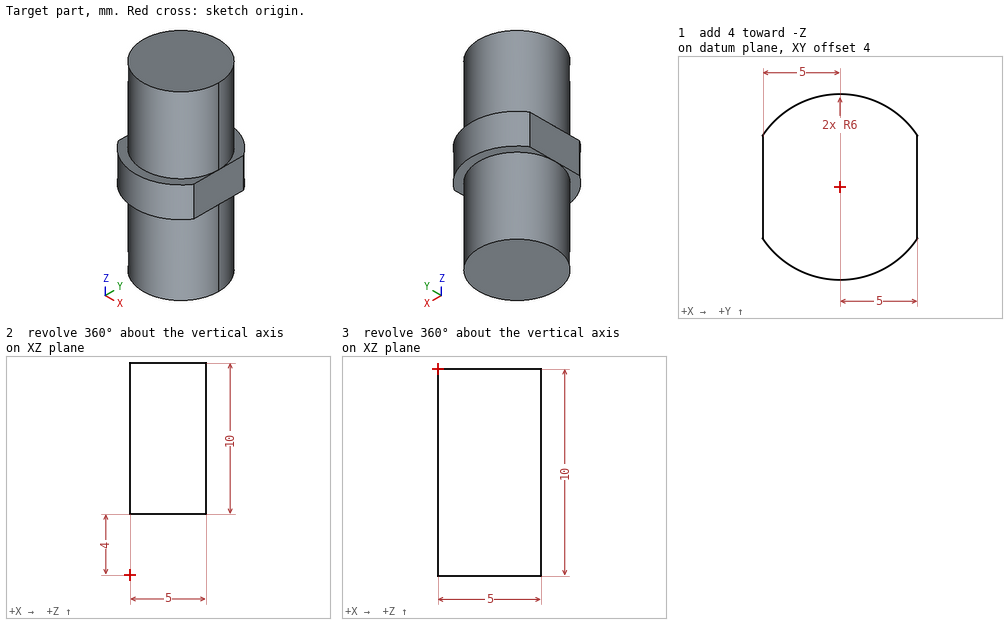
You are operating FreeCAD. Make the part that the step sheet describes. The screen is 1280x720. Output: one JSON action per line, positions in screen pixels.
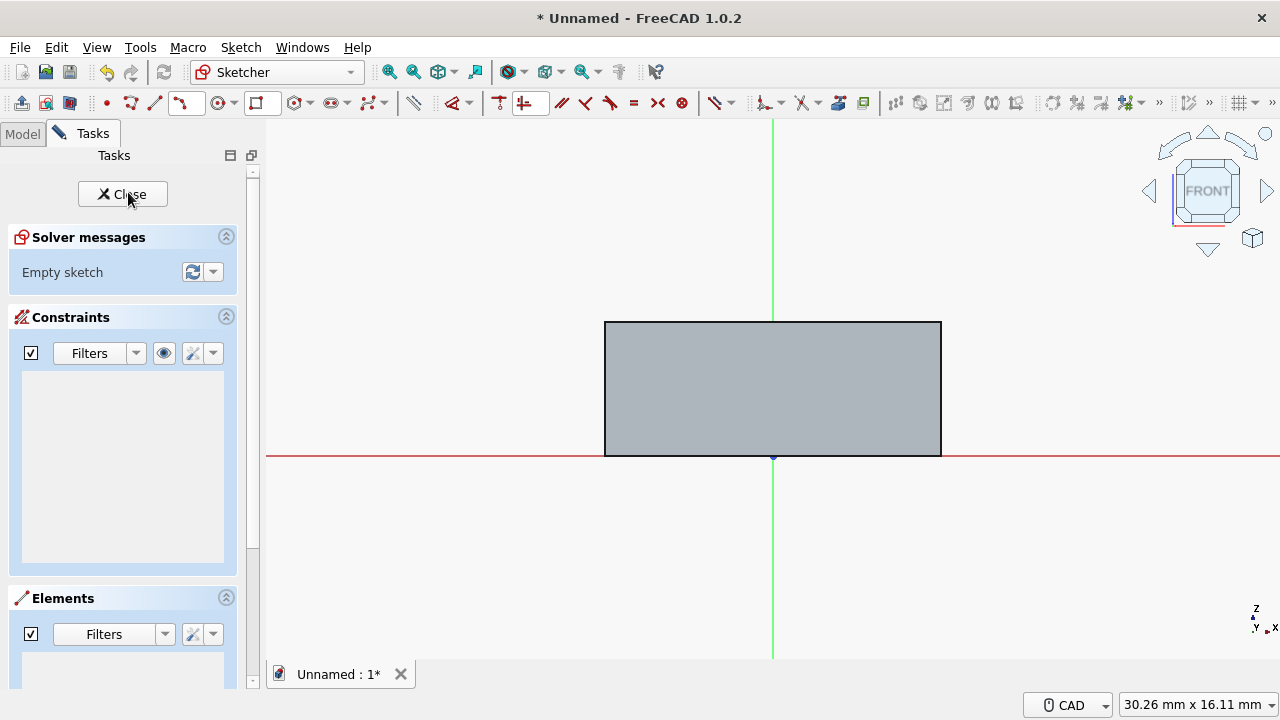
{"action": "left_click", "coordinate": [70, 104]}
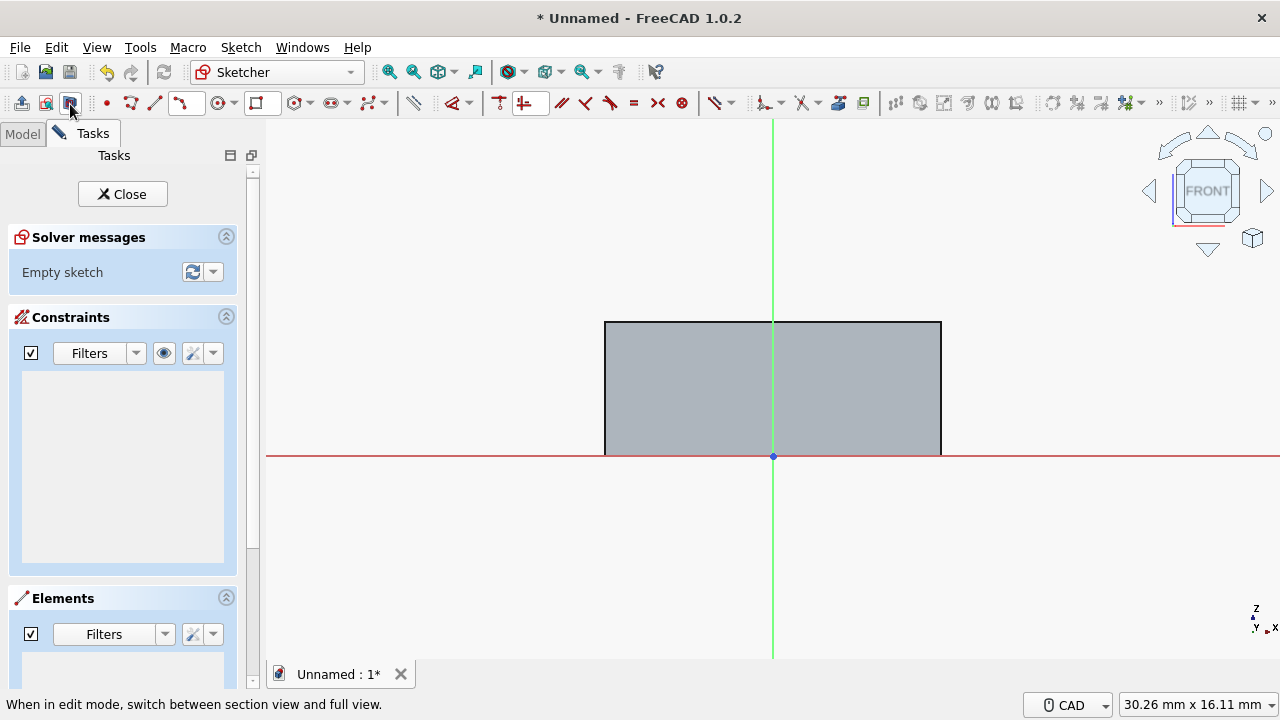
{"action": "scroll", "coordinate": [395, 631], "scroll_direction": "down", "scroll_amount": 2}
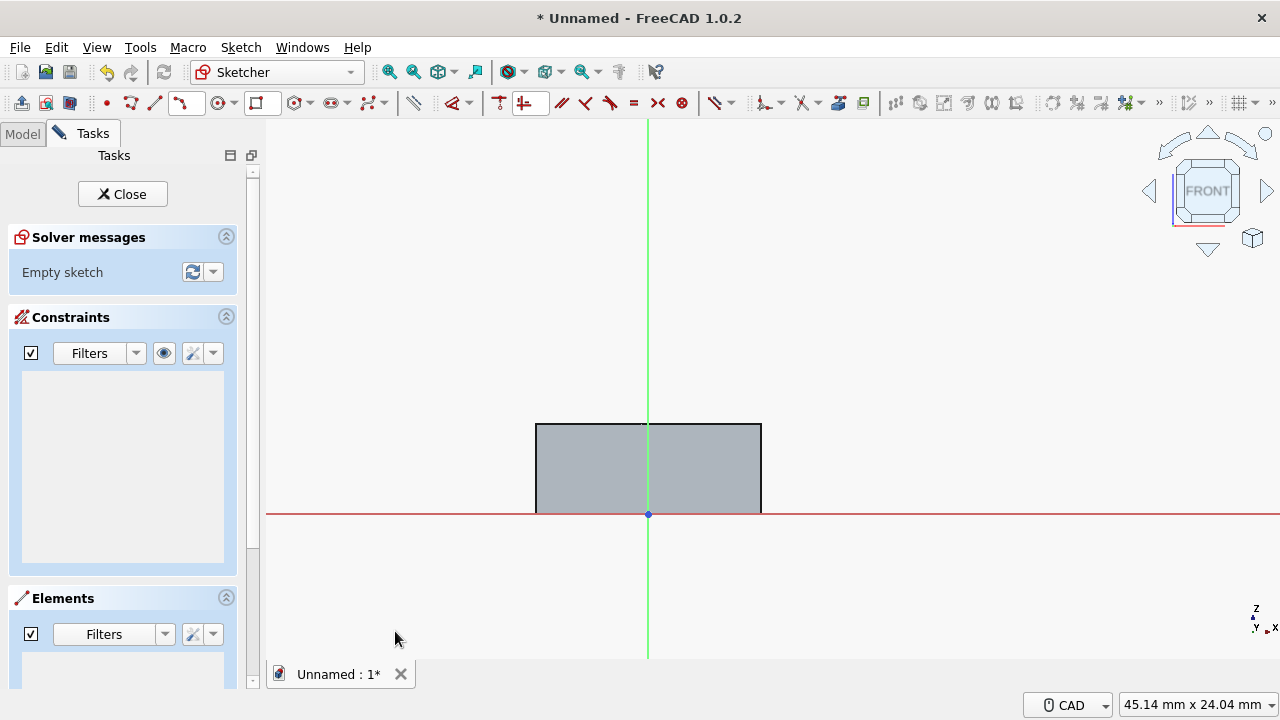
{"action": "left_click", "coordinate": [256, 104]}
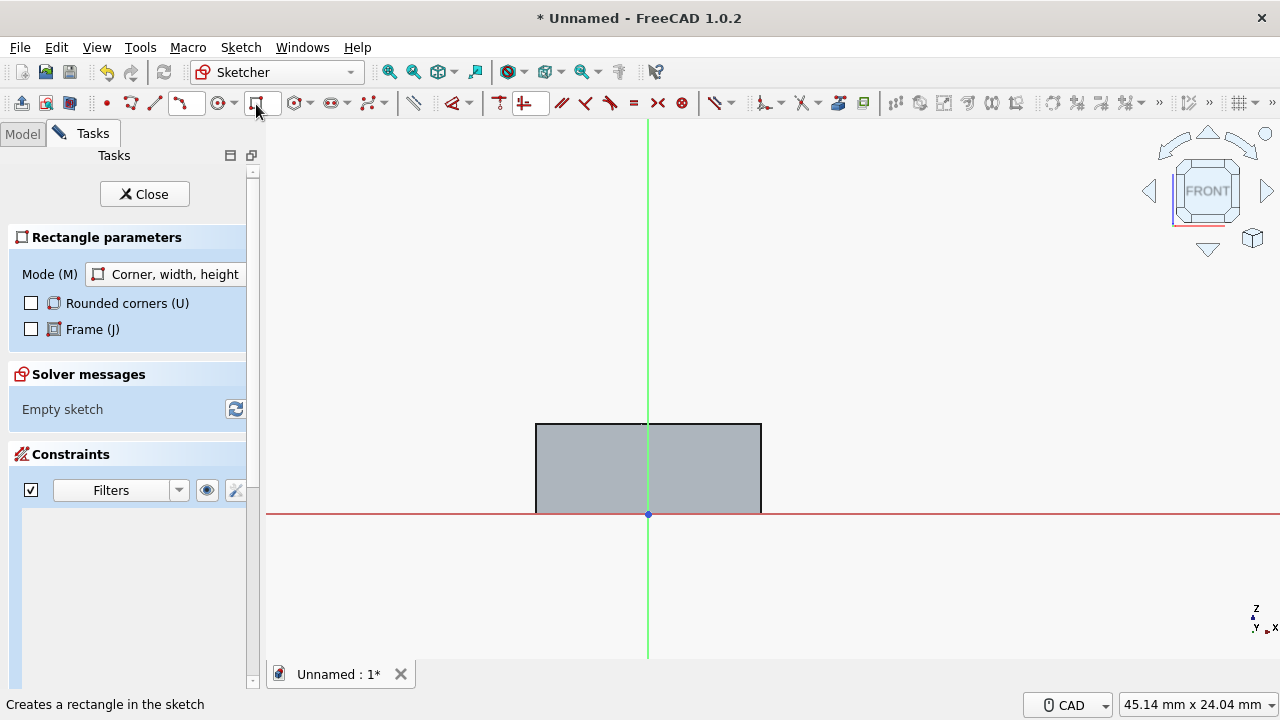
{"action": "left_click", "coordinate": [648, 200]}
{"action": "mouse_move", "coordinate": [761, 424]}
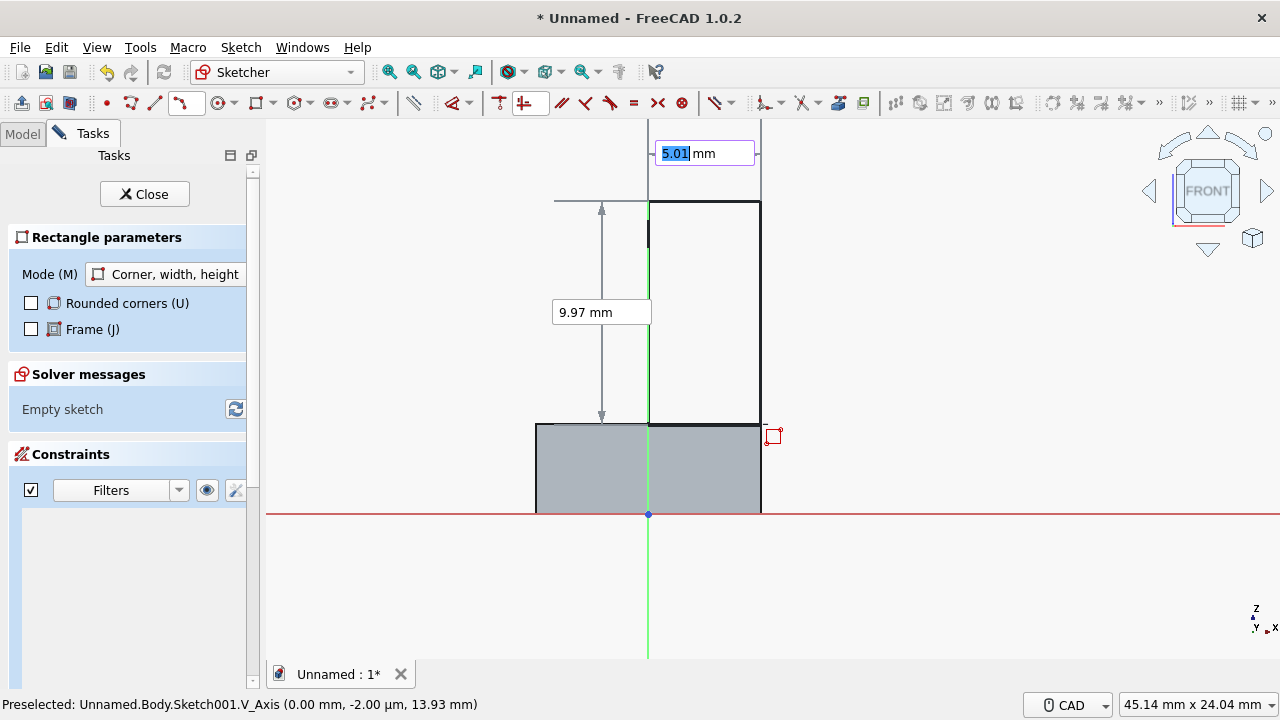
{"action": "type", "text": "5"}
{"action": "key", "text": "Tab"}
{"action": "type", "text": "10"}
{"action": "key", "text": "Return"}
{"action": "key", "text": "Escape"}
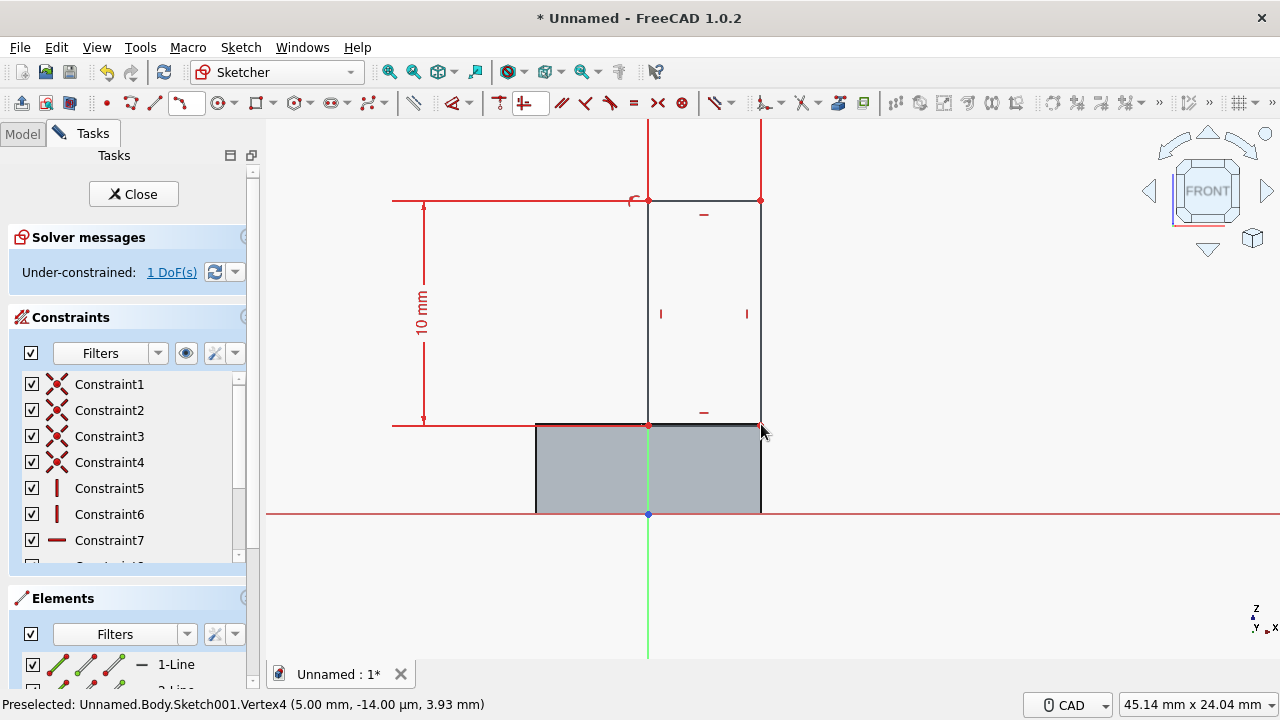
{"action": "left_click", "coordinate": [452, 104]}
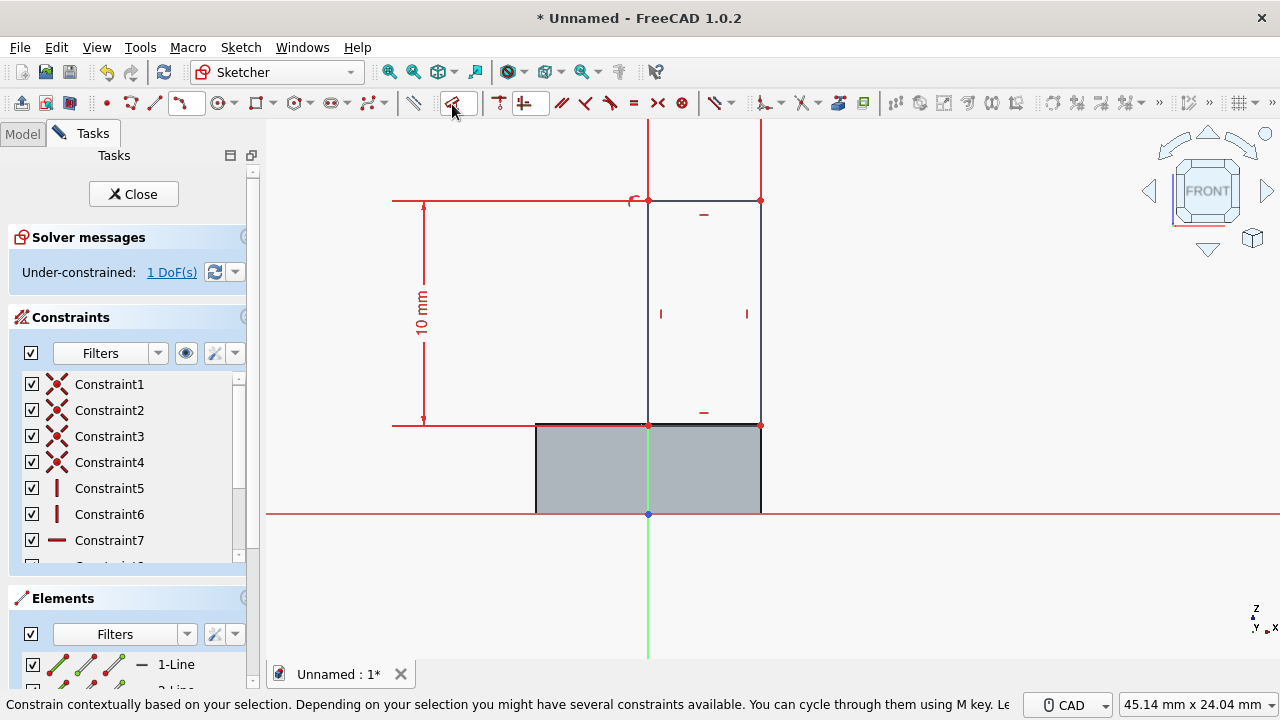
{"action": "left_click", "coordinate": [648, 426]}
{"action": "left_click", "coordinate": [614, 470]}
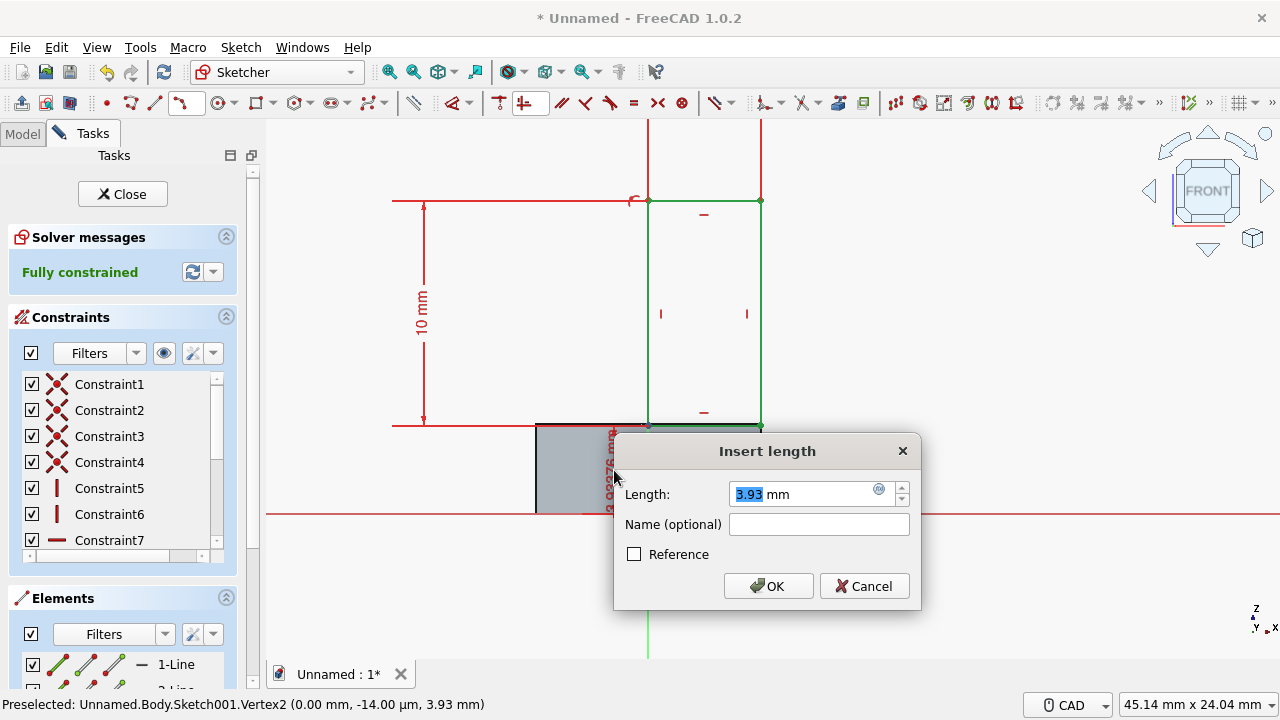
{"action": "type", "text": "4"}
{"action": "key", "text": "Return"}
{"action": "key", "text": "Escape"}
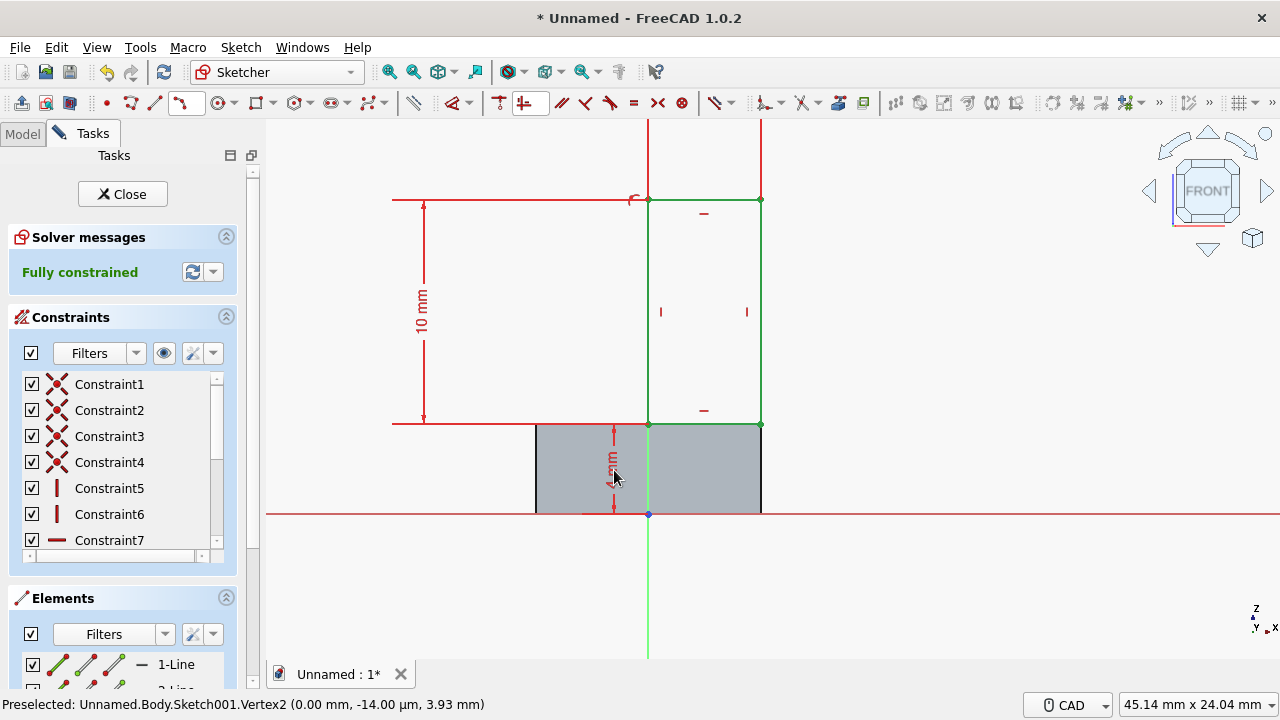
{"action": "left_click", "coordinate": [123, 194]}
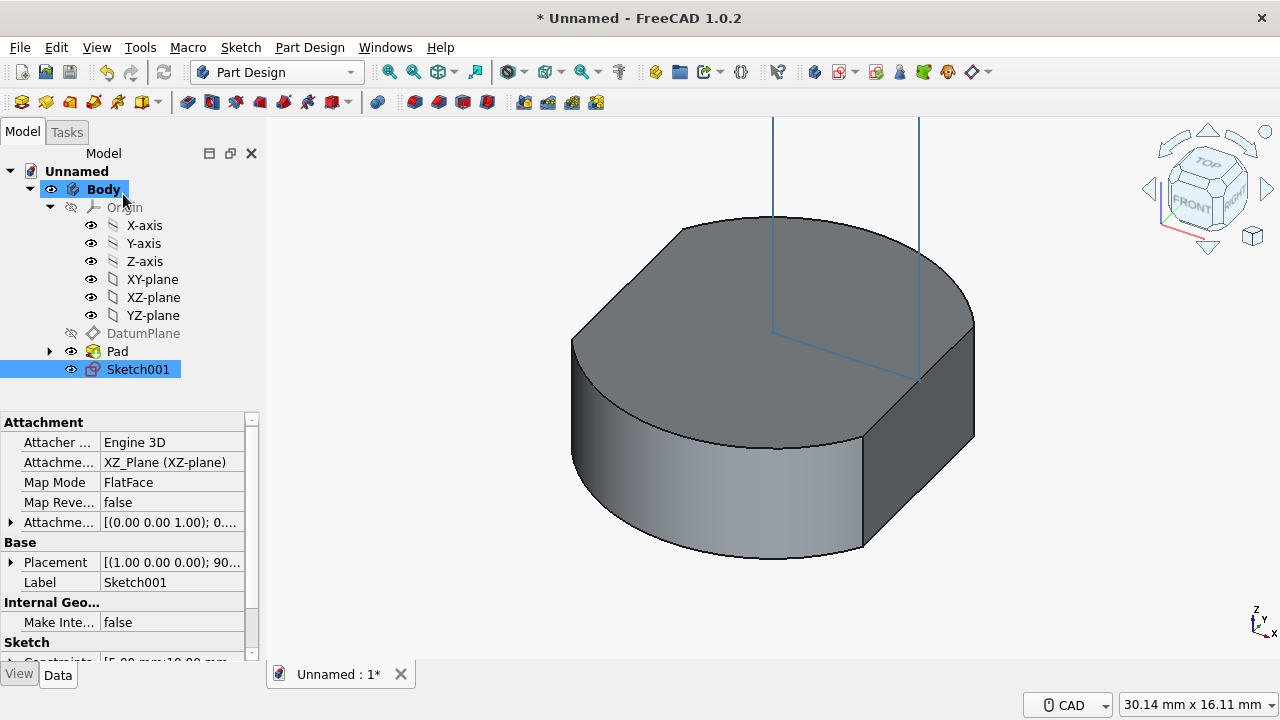
{"action": "left_click", "coordinate": [46, 102]}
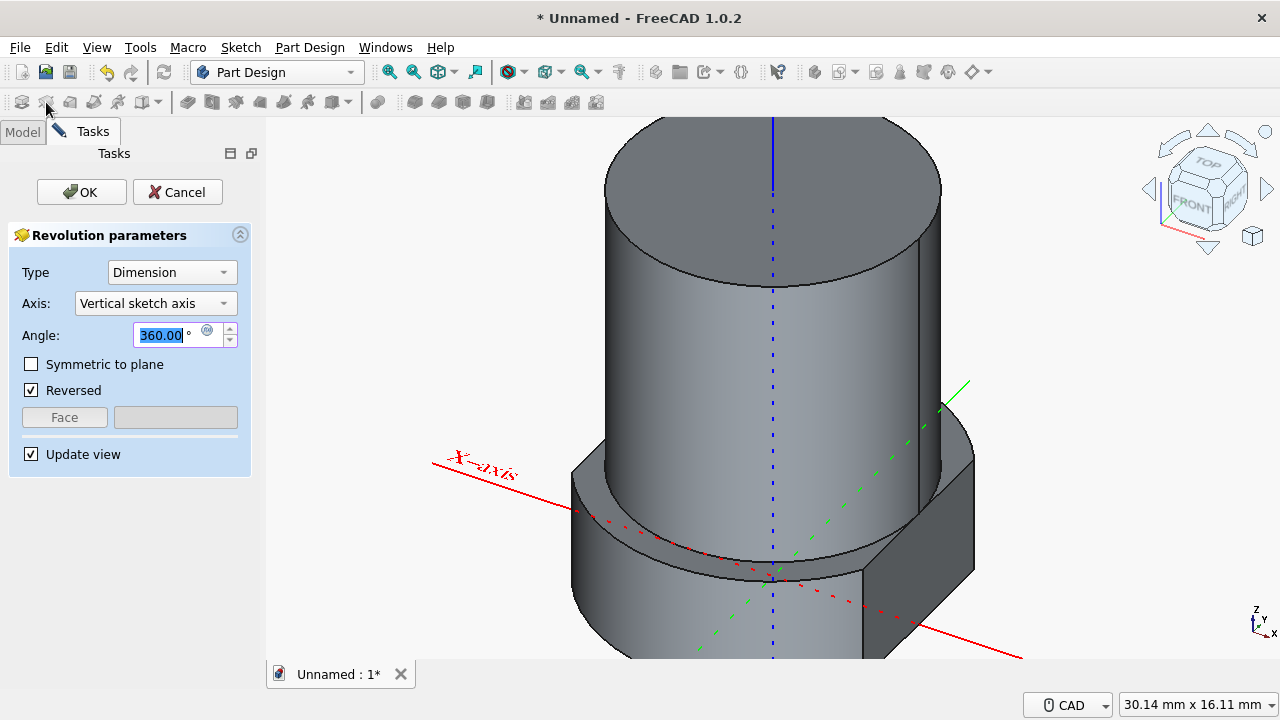
{"action": "left_click", "coordinate": [82, 192]}